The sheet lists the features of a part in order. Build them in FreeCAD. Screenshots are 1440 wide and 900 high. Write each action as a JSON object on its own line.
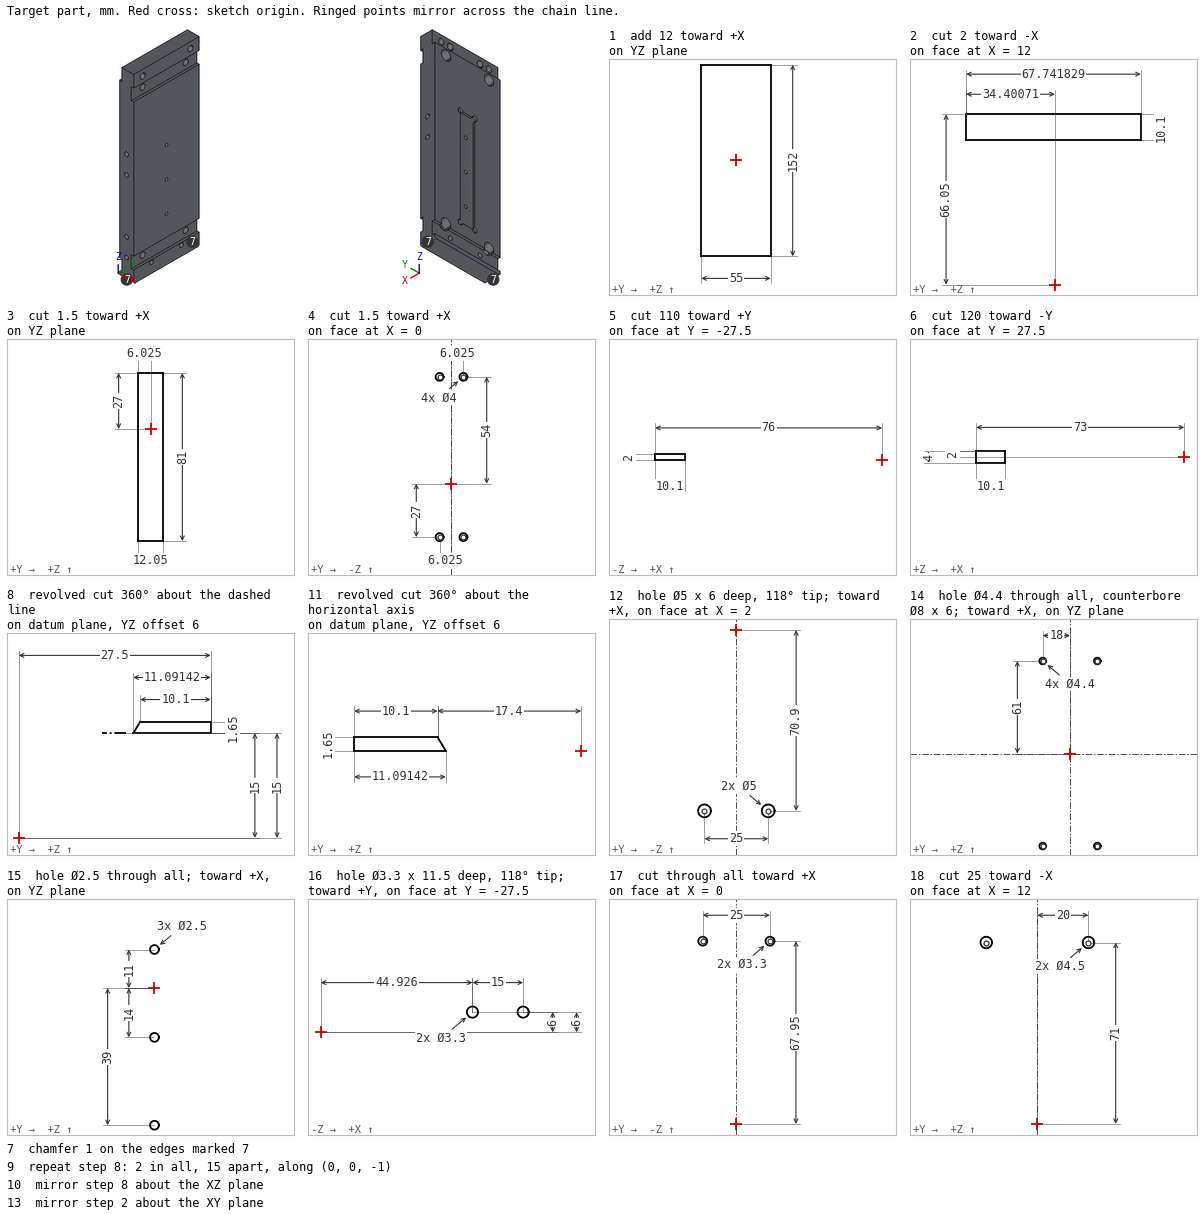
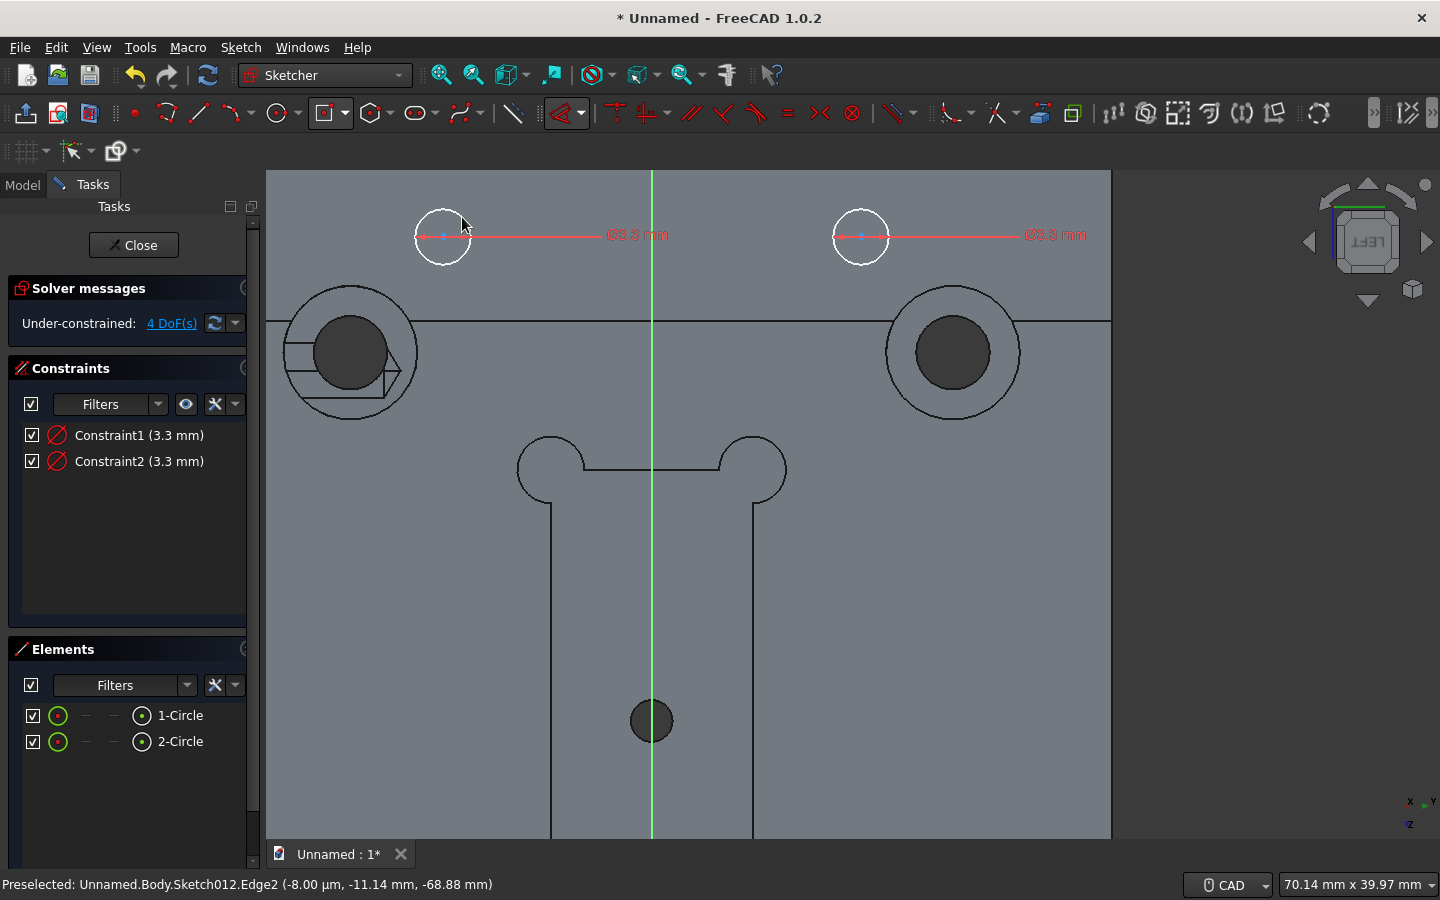
{"action": "left_click", "coordinate": [861, 237]}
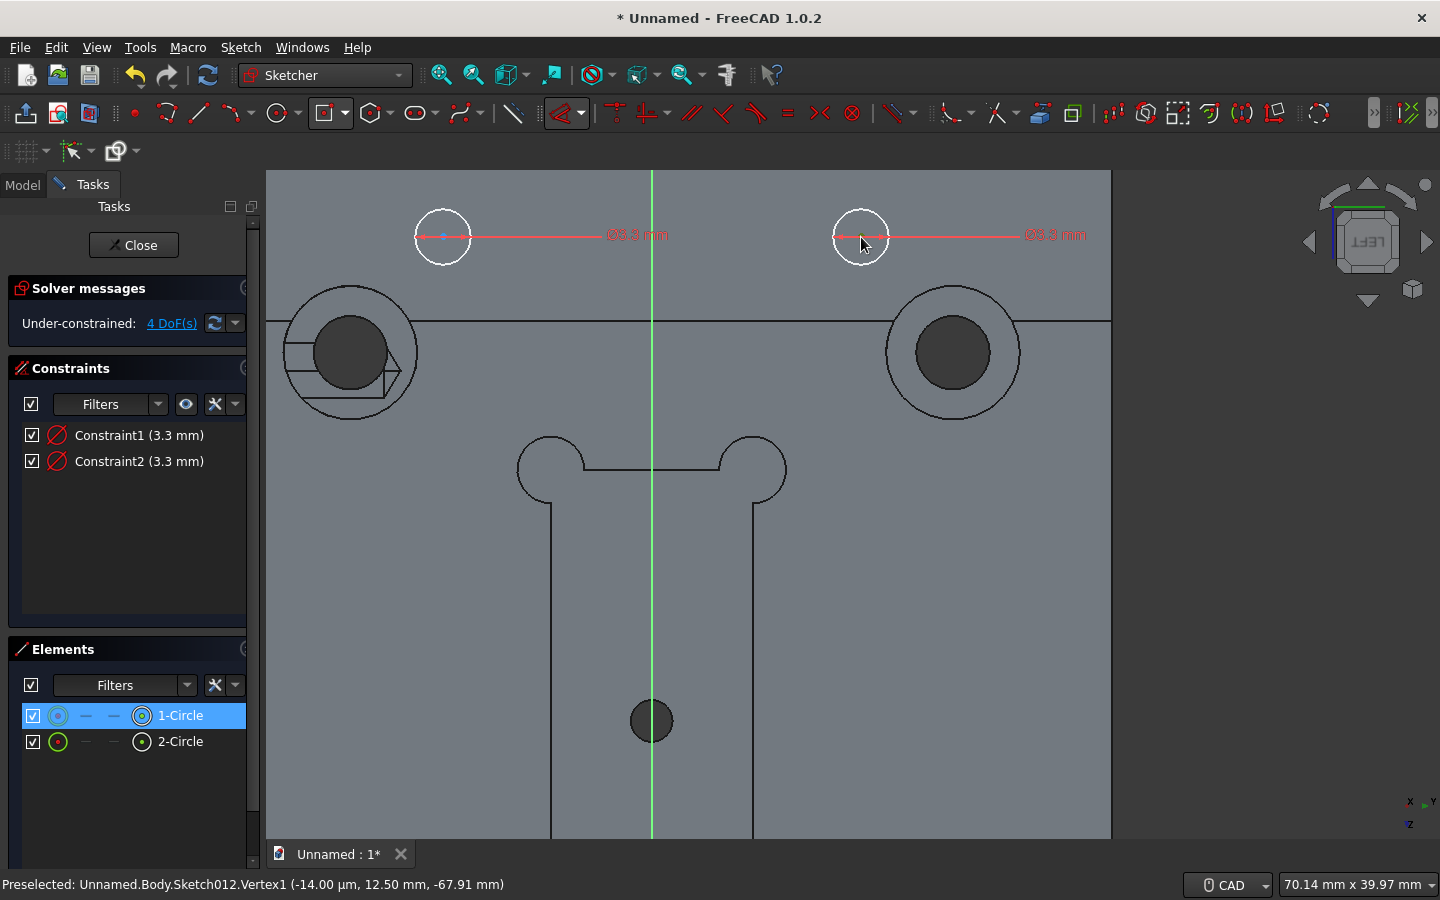
{"action": "left_click", "coordinate": [443, 237]}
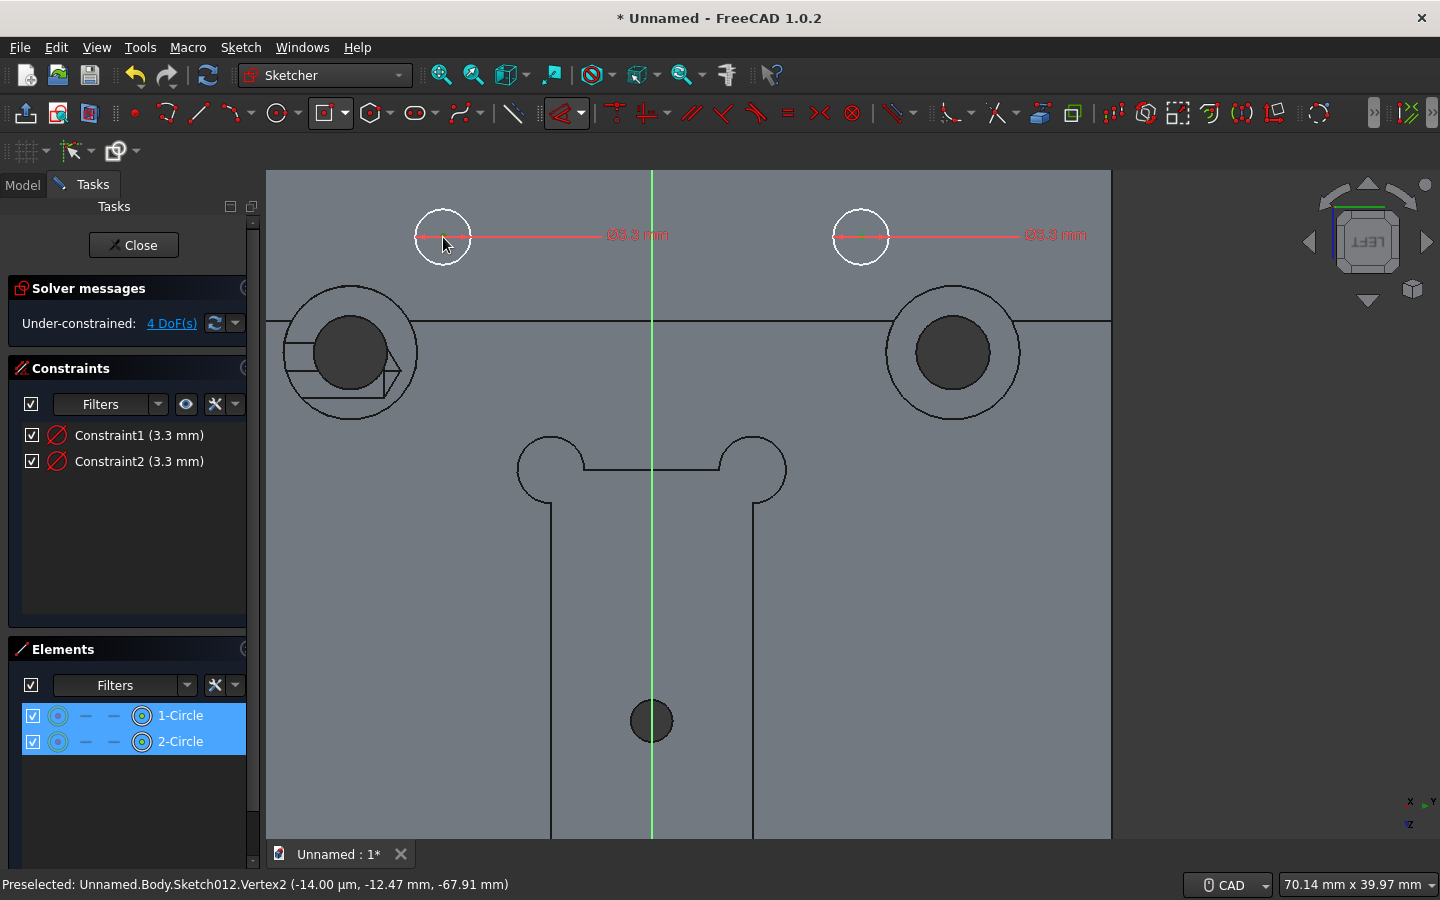
{"action": "left_click", "coordinate": [652, 767]}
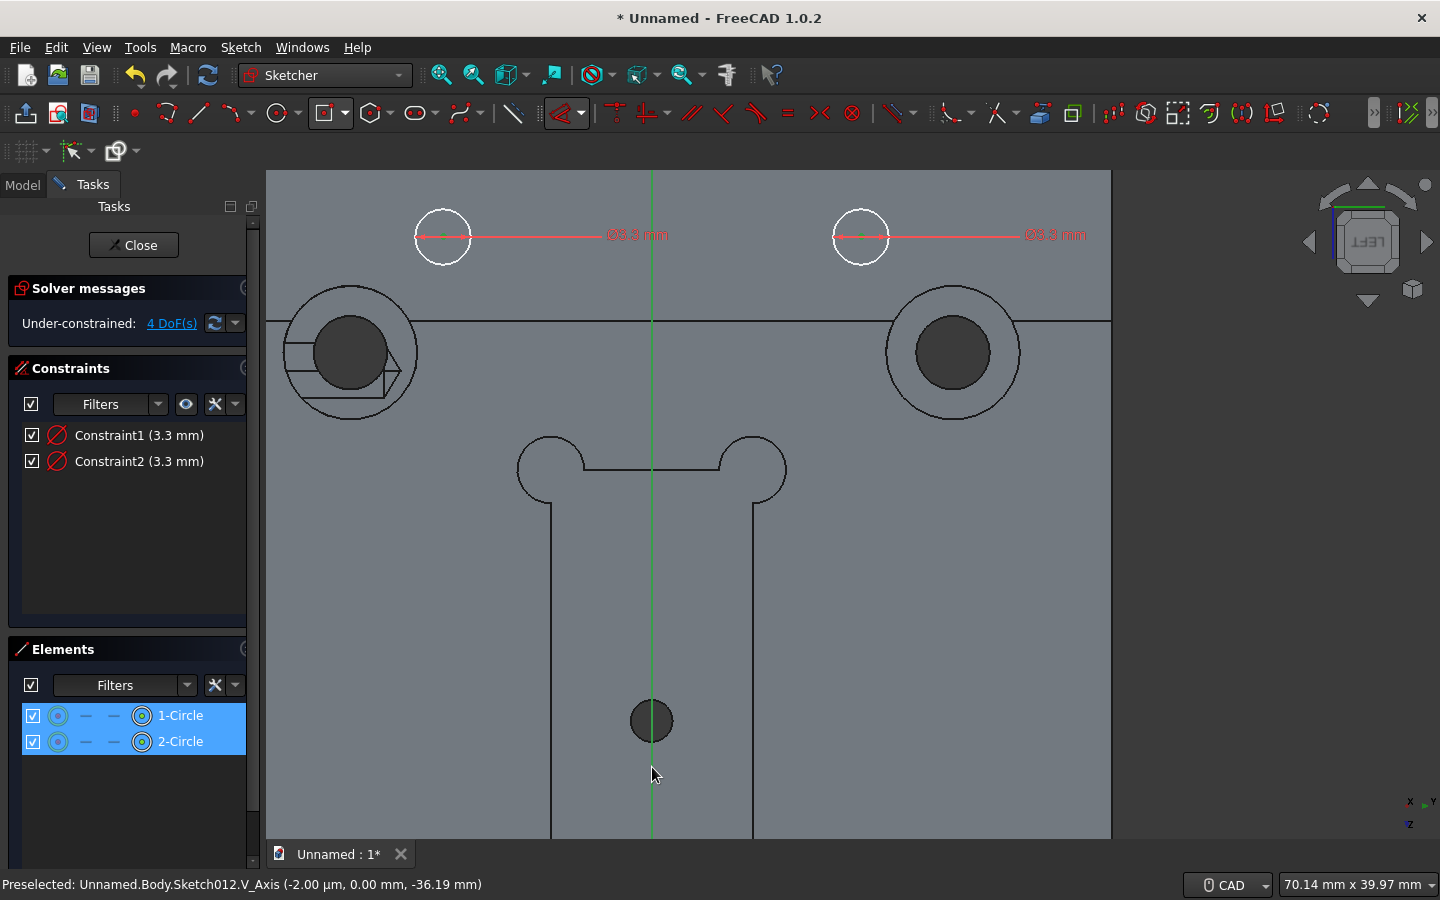
{"action": "left_click", "coordinate": [820, 114]}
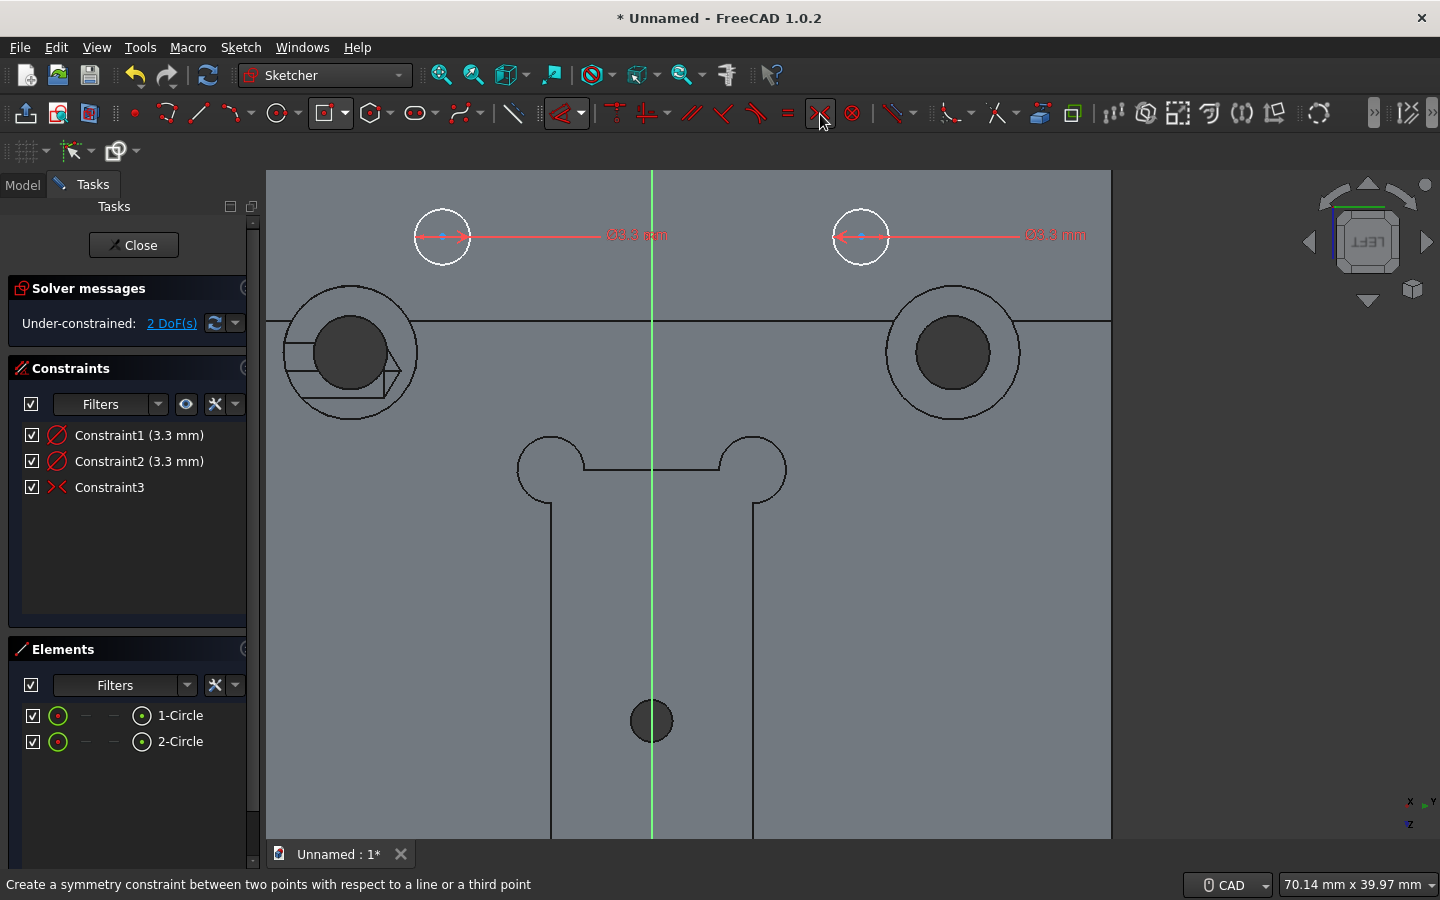
{"action": "left_click", "coordinate": [861, 237]}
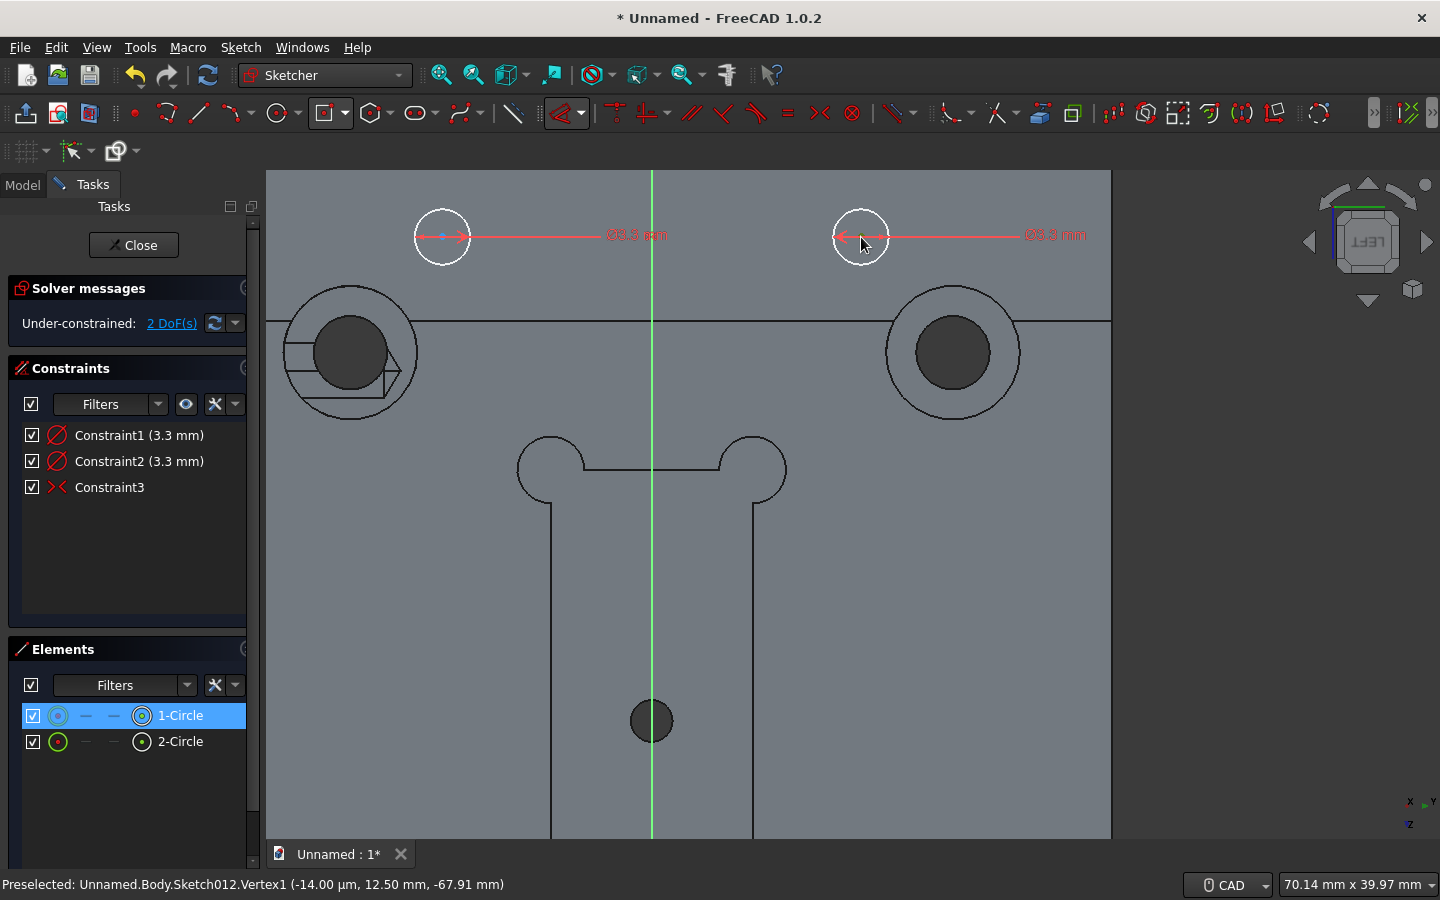
{"action": "left_click", "coordinate": [442, 237]}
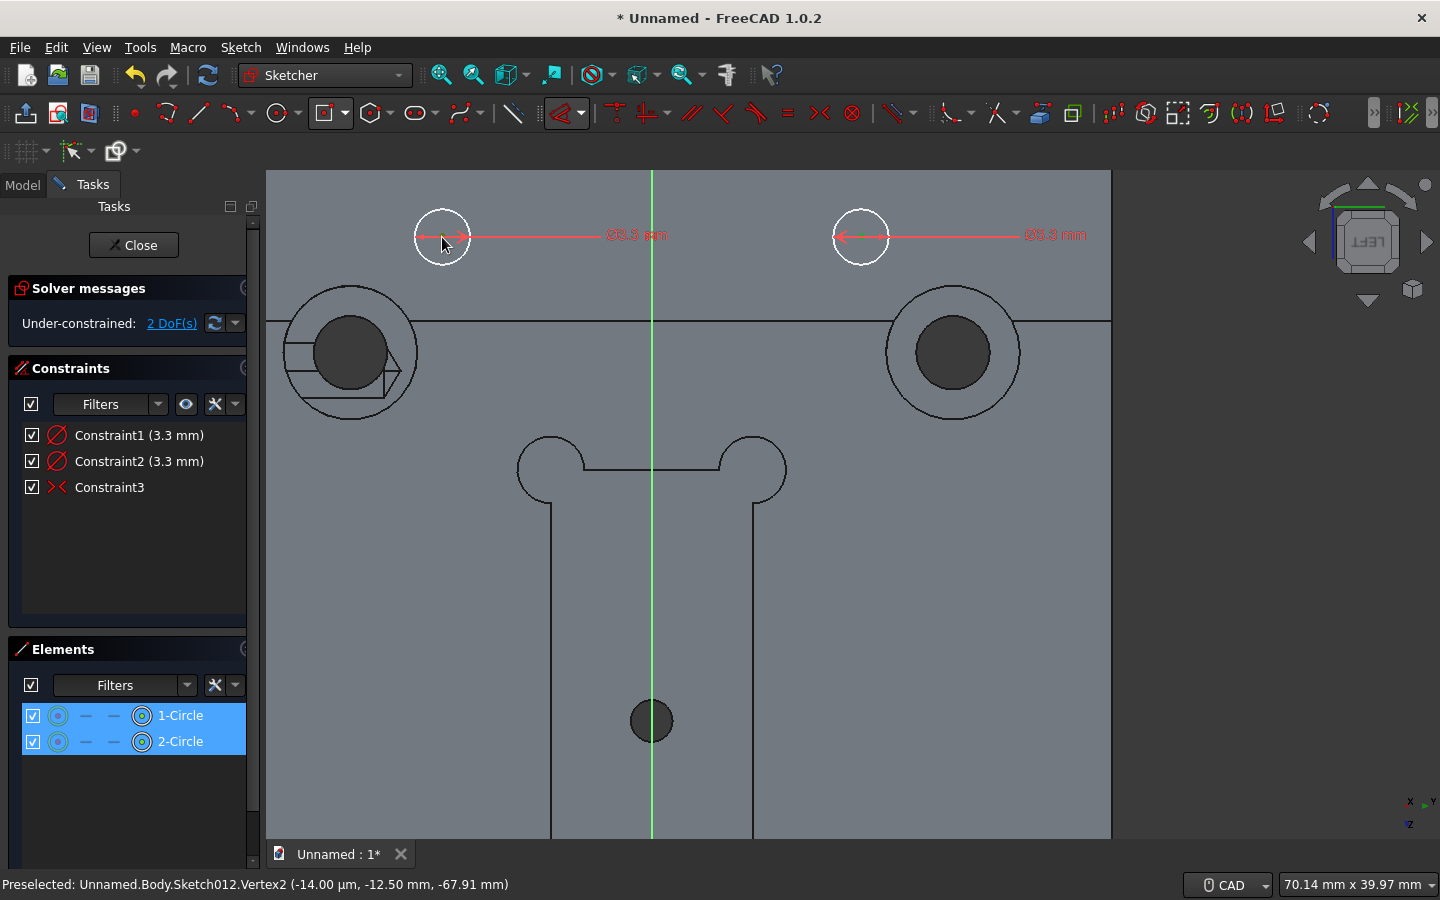
{"action": "key", "text": "l"}